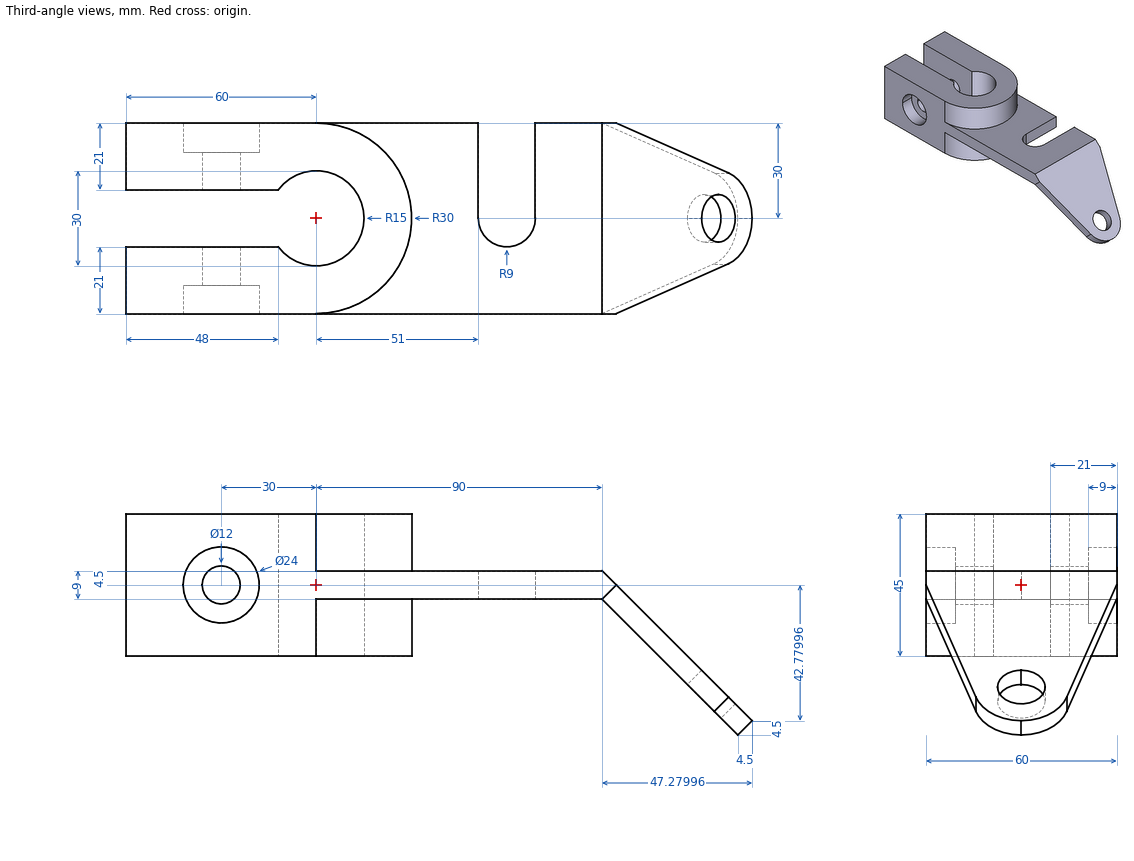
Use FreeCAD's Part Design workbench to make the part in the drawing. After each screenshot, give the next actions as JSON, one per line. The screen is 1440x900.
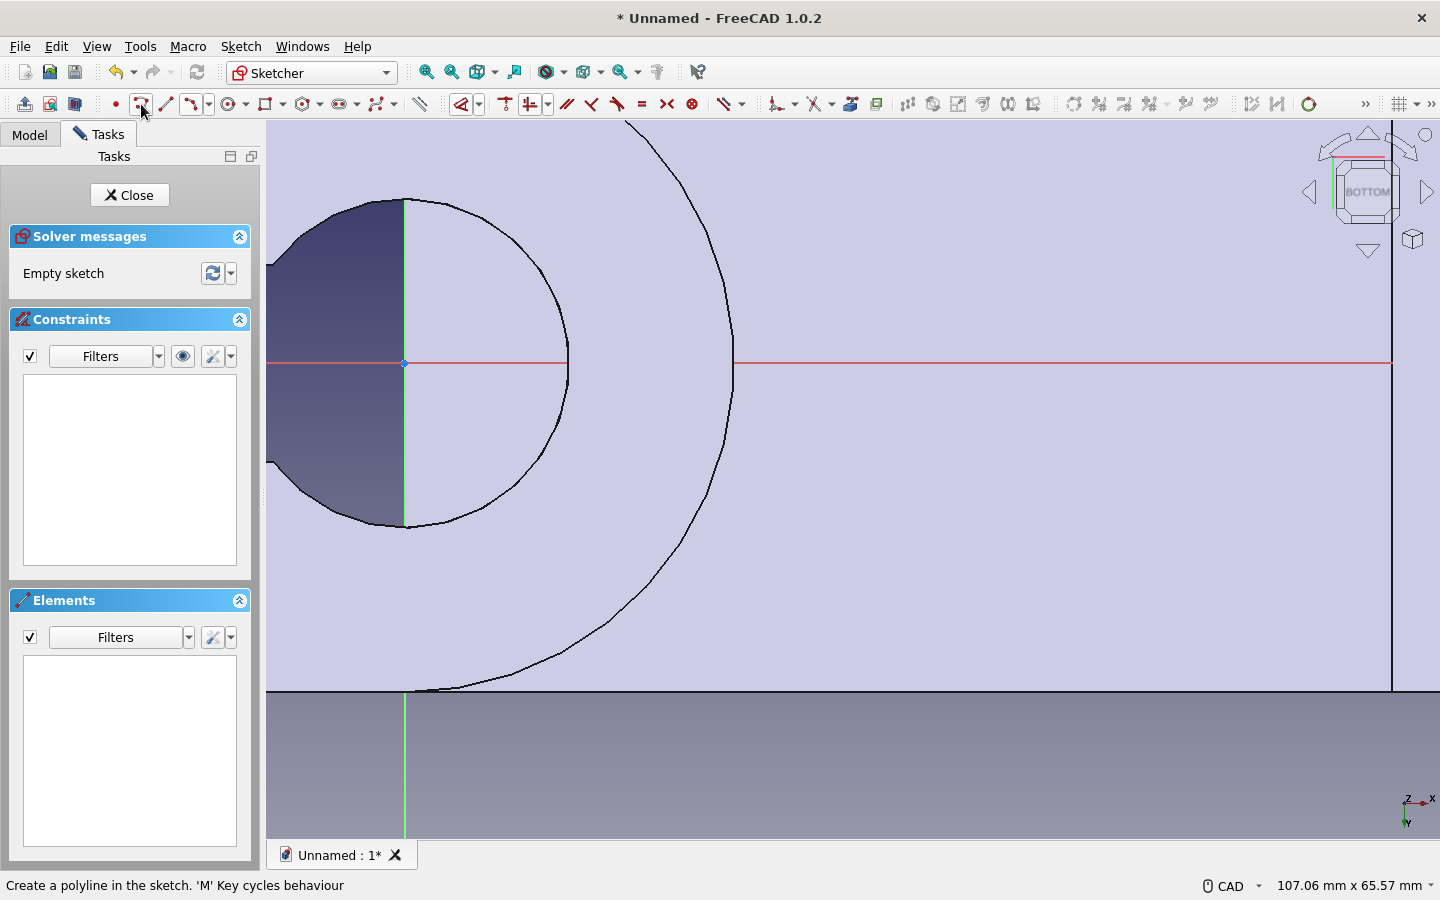
{"action": "left_click", "coordinate": [964, 363]}
{"action": "left_click", "coordinate": [964, 692]}
{"action": "left_click", "coordinate": [1162, 692]}
{"action": "left_click", "coordinate": [1162, 363]}
{"action": "right_click", "coordinate": [1162, 363]}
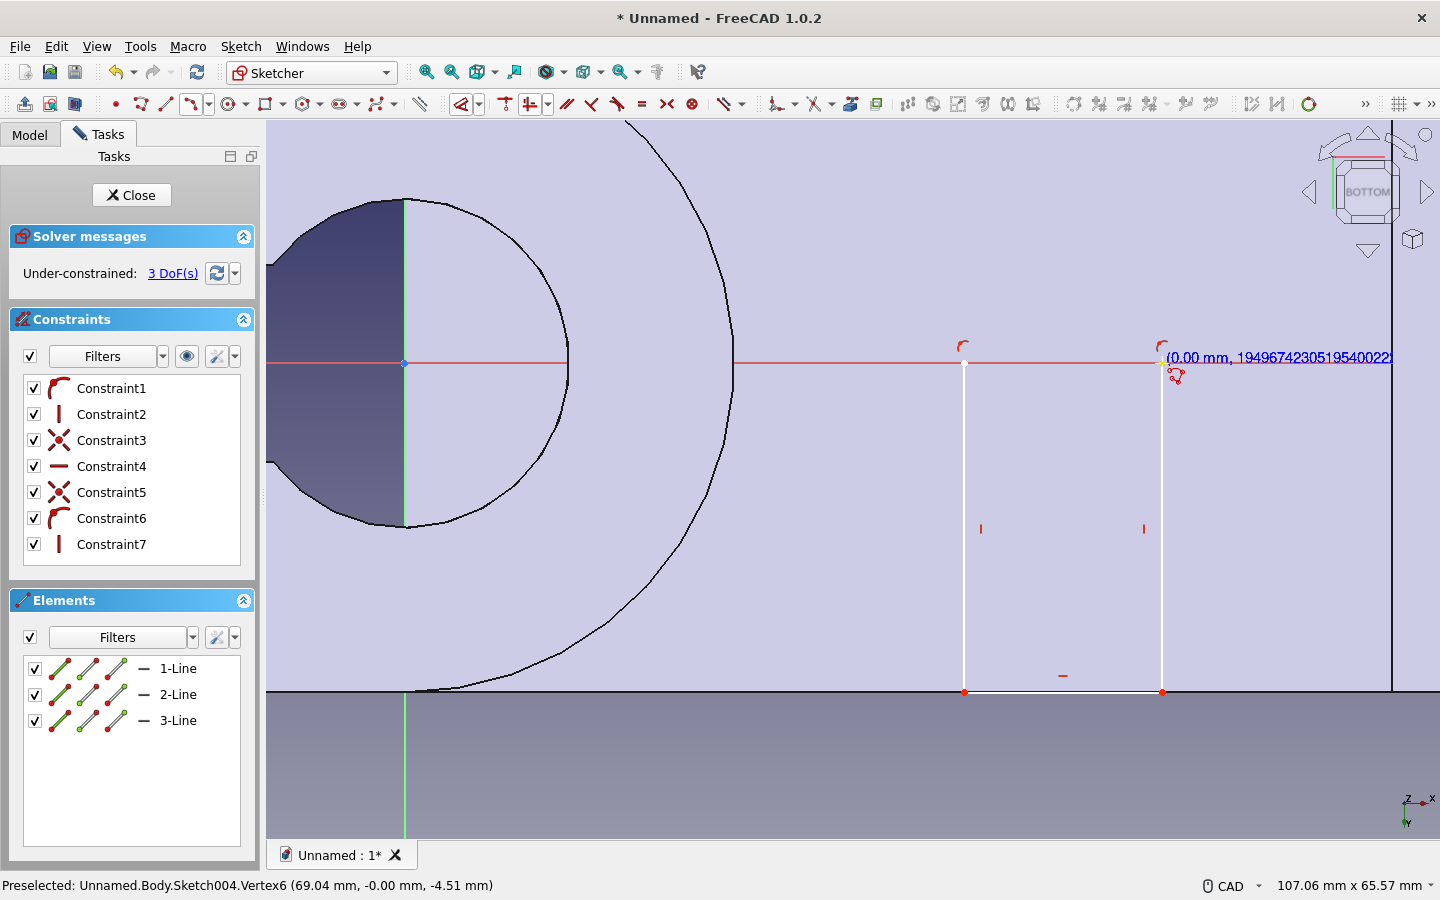
{"action": "key", "text": "g 3 a"}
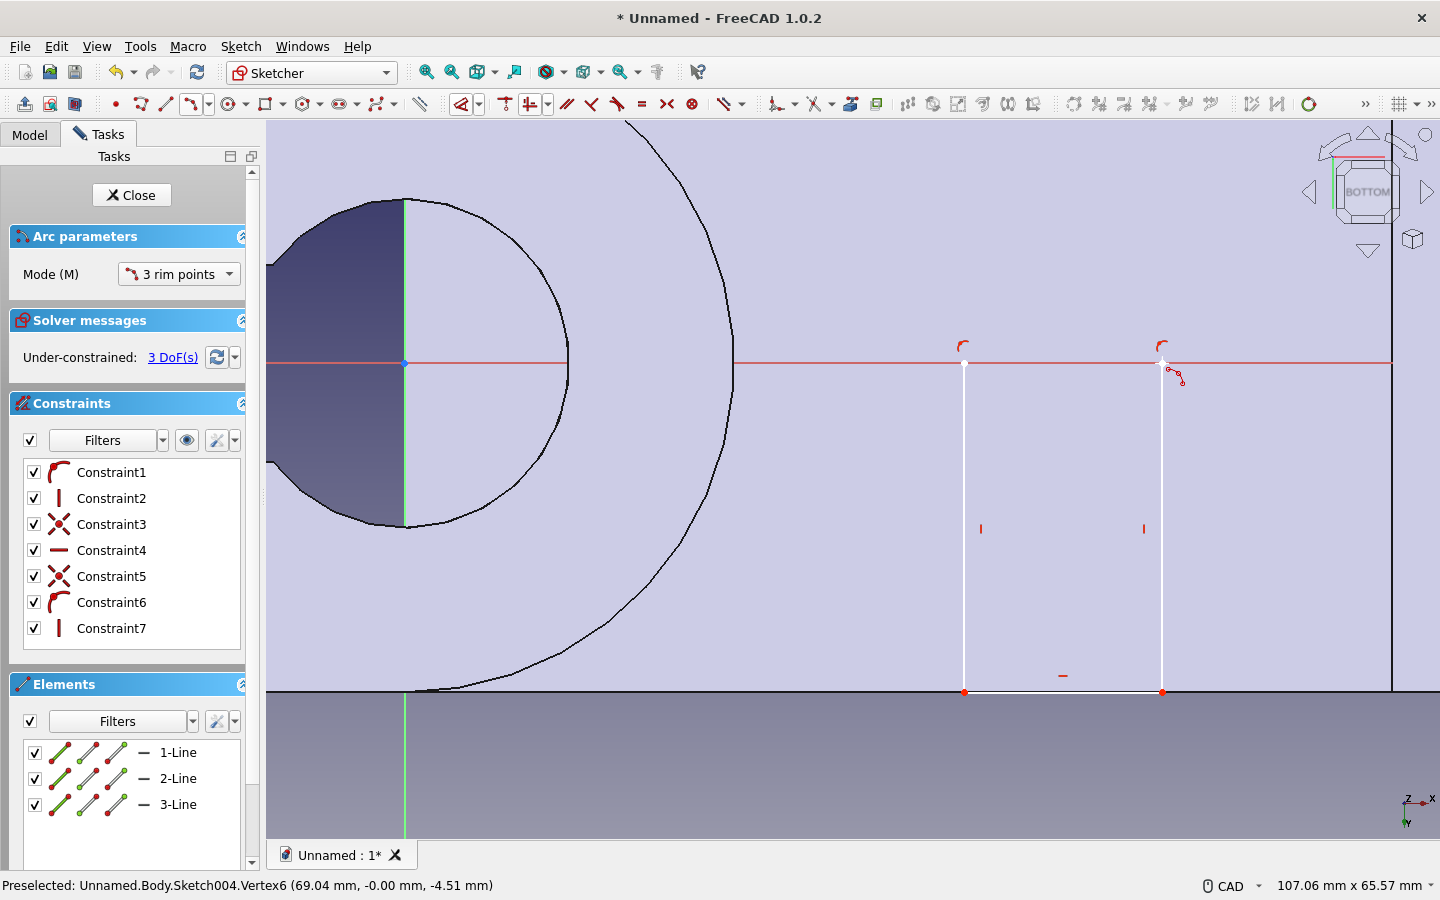
{"action": "left_click", "coordinate": [1162, 363]}
{"action": "left_click", "coordinate": [964, 363]}
{"action": "left_click", "coordinate": [1063, 265]}
{"action": "key", "text": "Escape"}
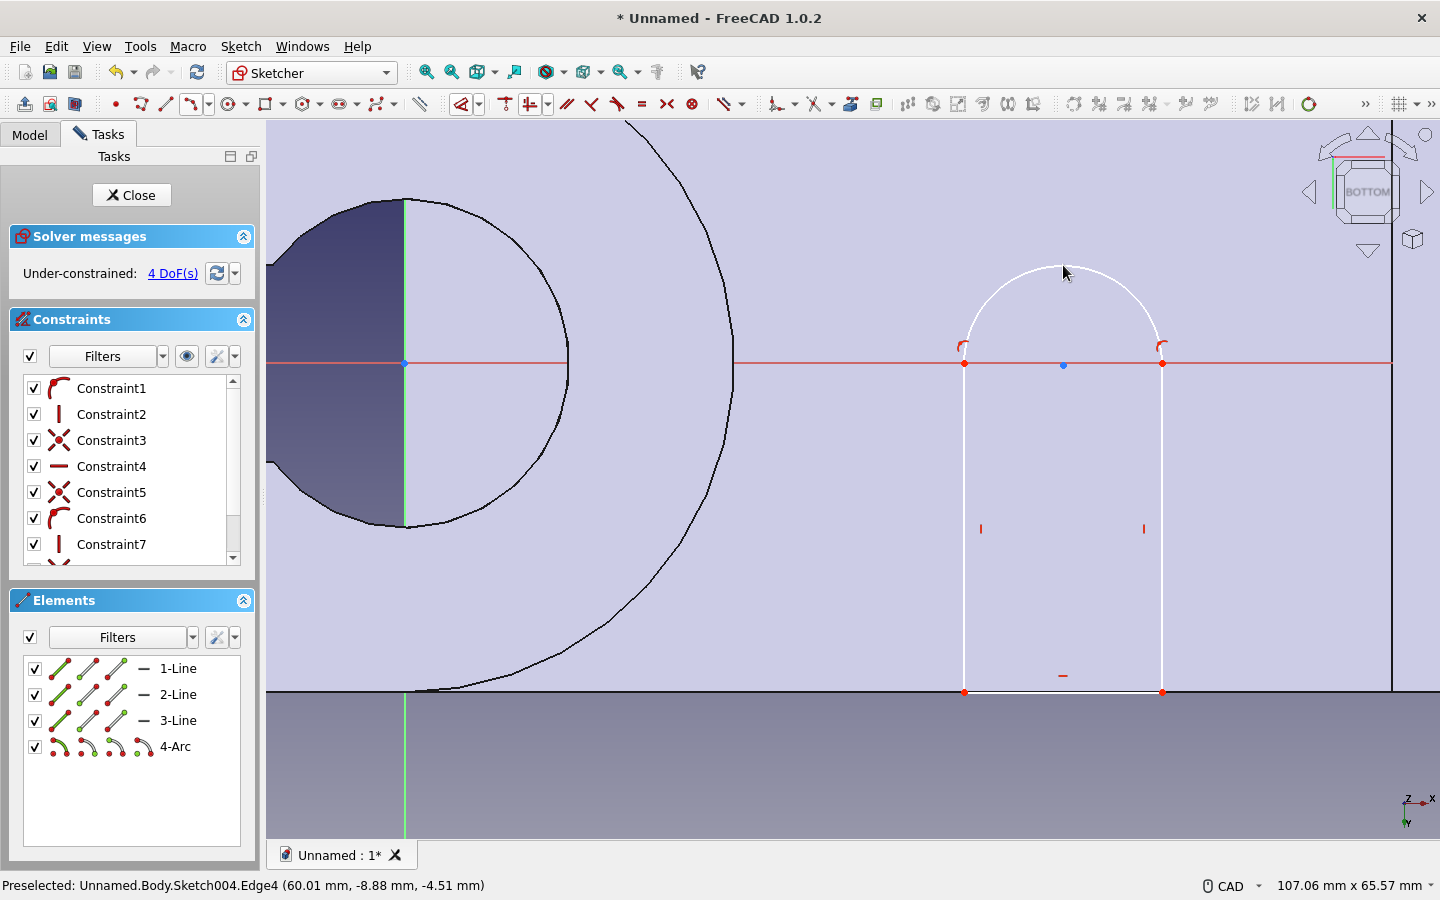
{"action": "left_click", "coordinate": [964, 462]}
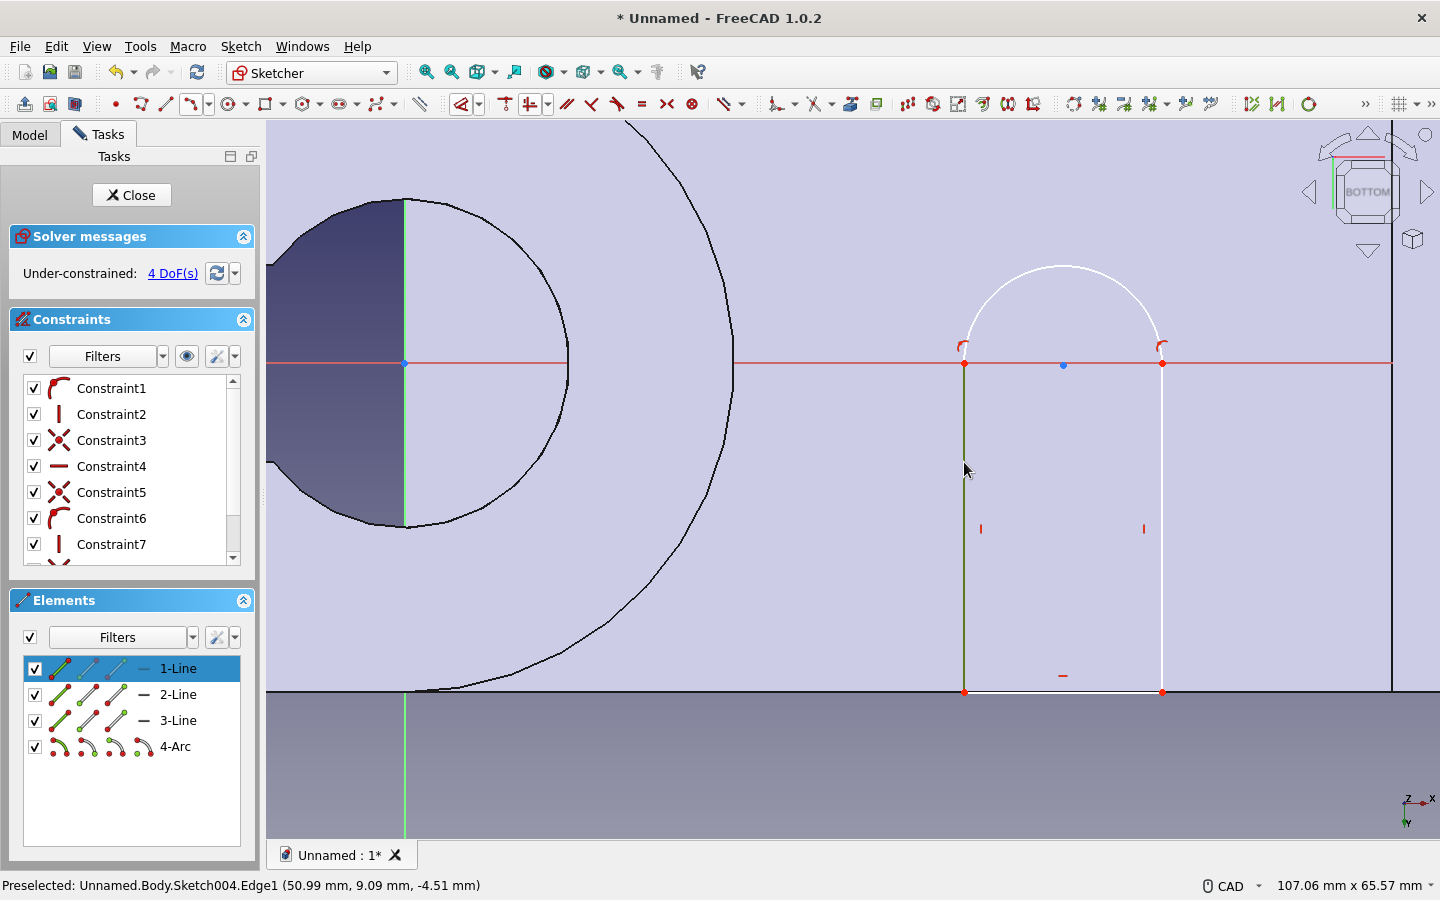
{"action": "left_click", "coordinate": [1121, 285]}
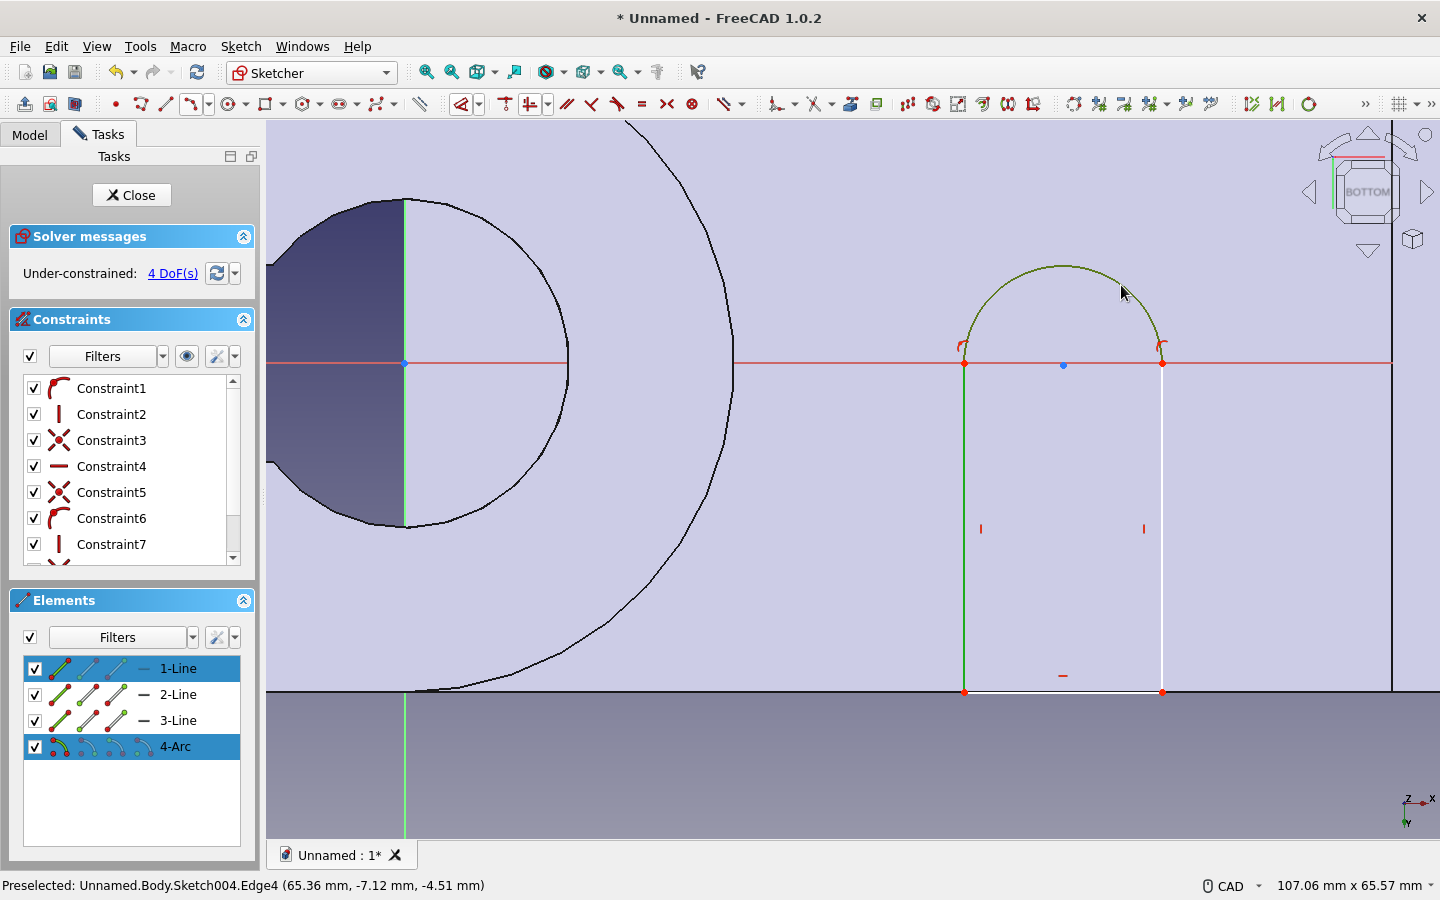
{"action": "left_click", "coordinate": [617, 104]}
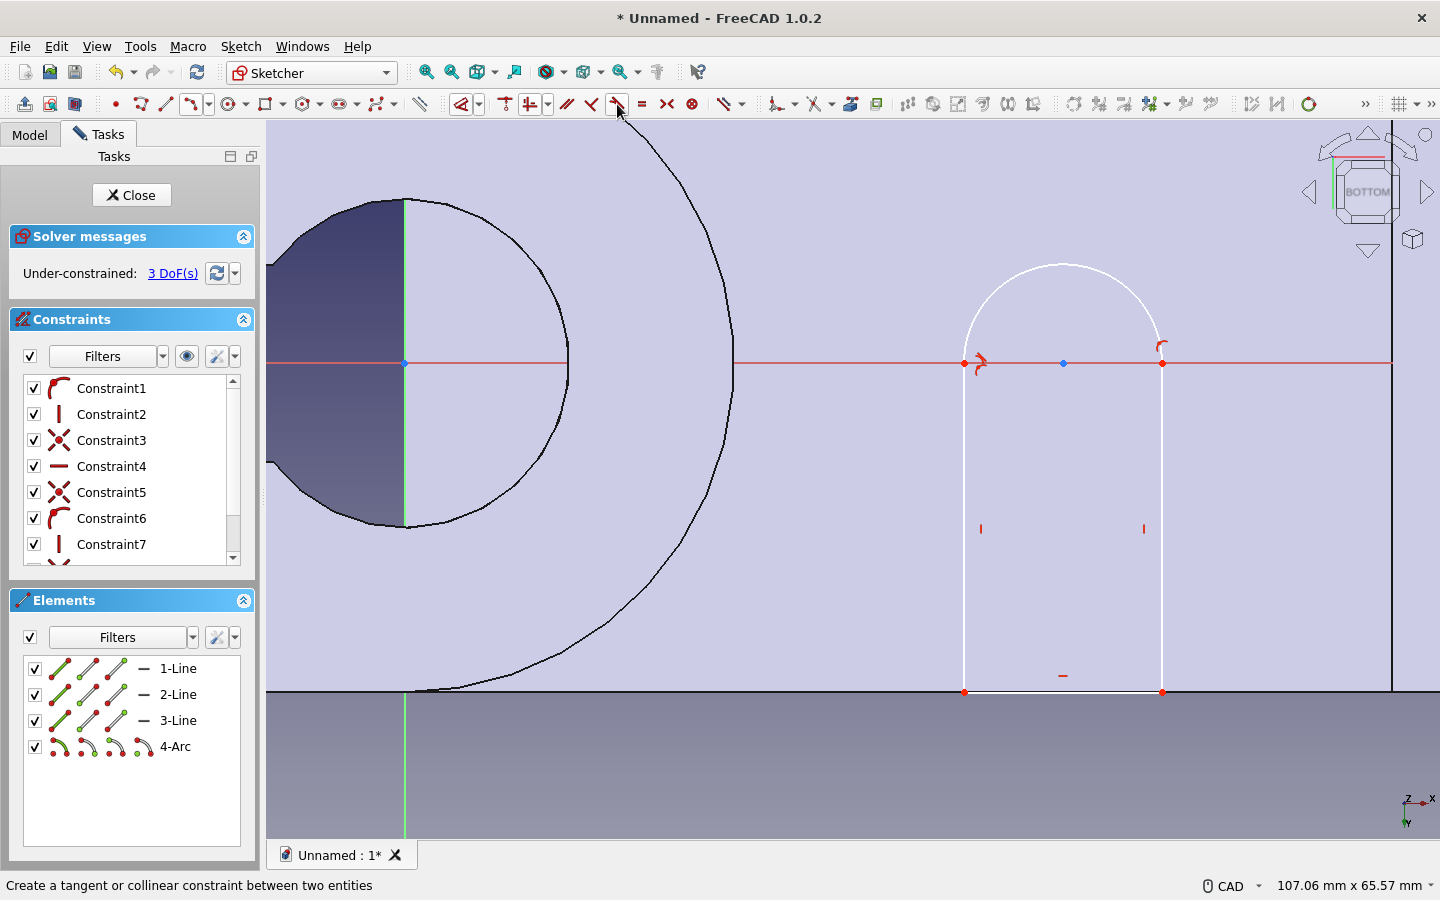
{"action": "left_click", "coordinate": [1121, 283]}